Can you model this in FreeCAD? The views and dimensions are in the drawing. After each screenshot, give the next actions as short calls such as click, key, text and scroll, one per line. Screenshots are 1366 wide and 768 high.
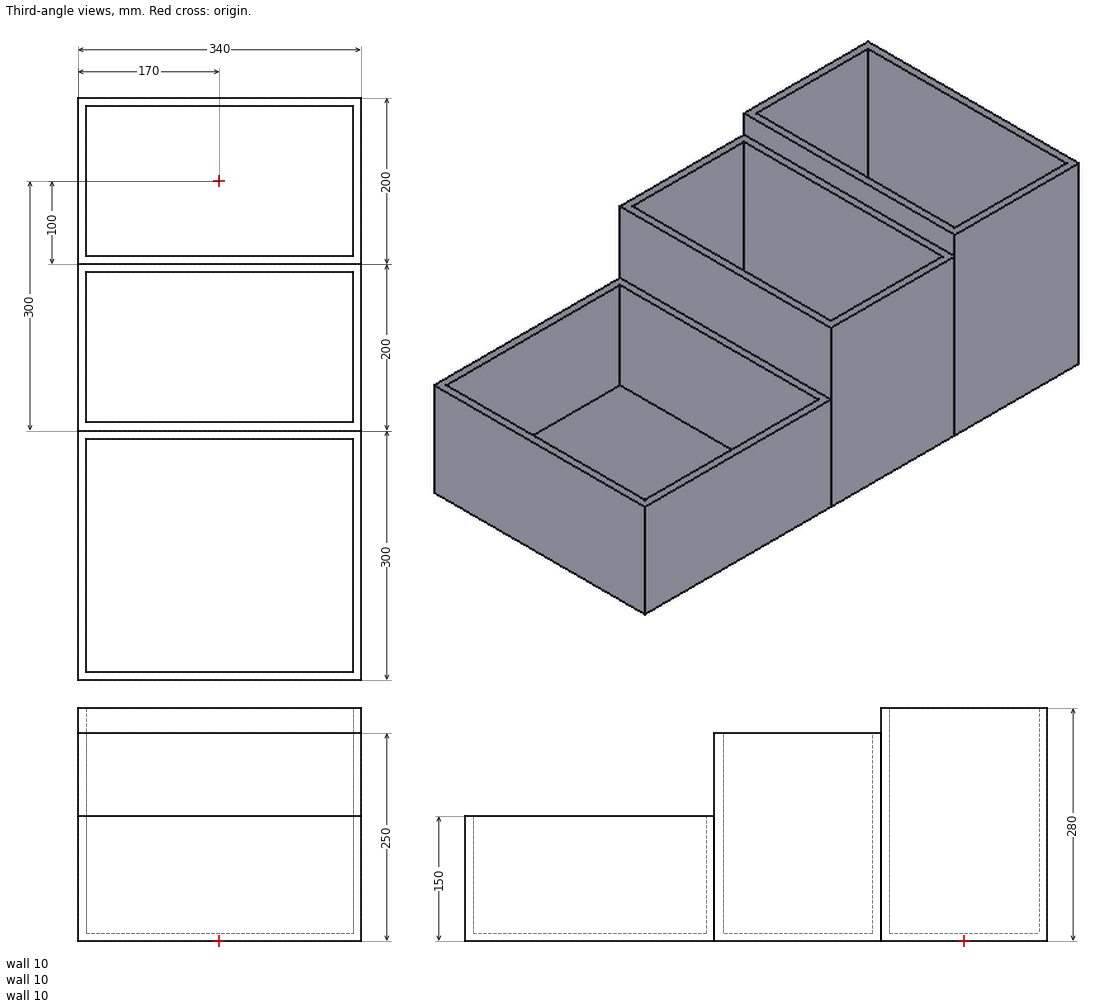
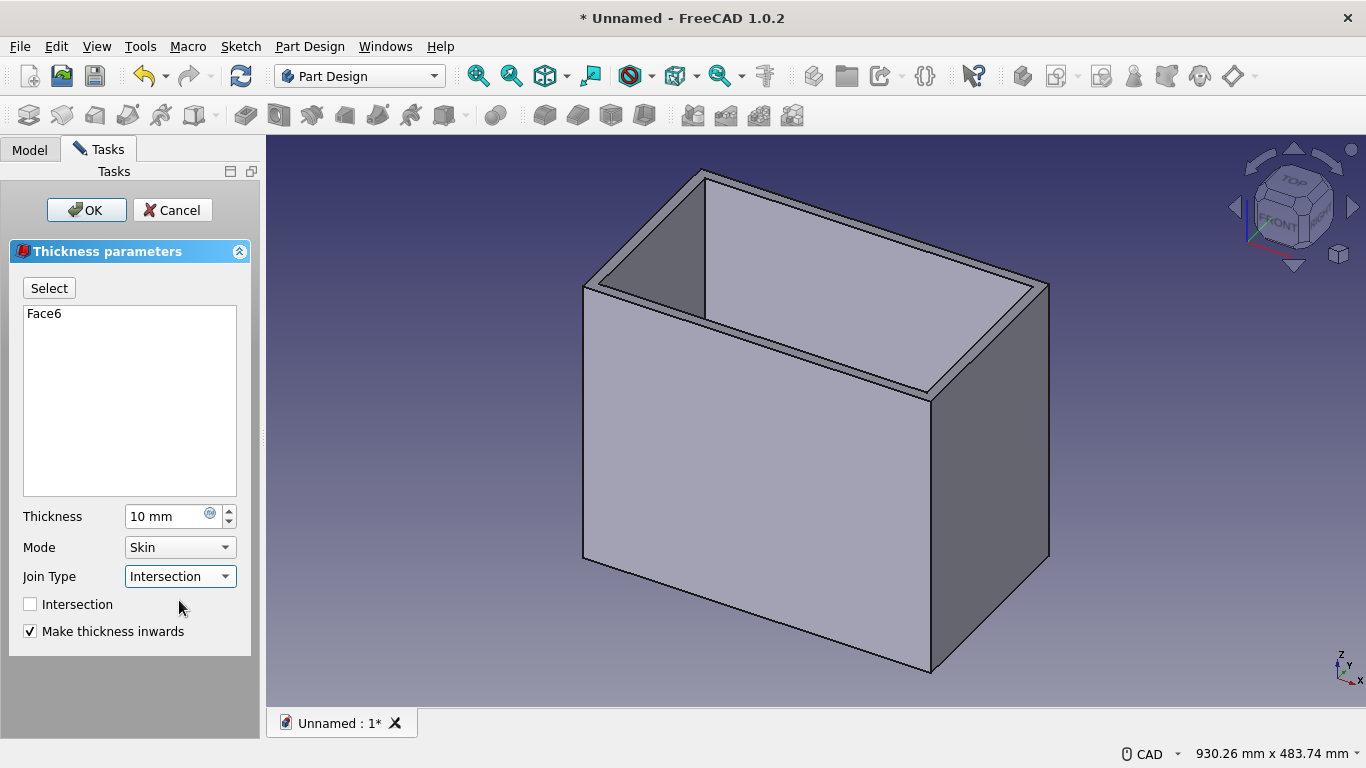
click(87, 210)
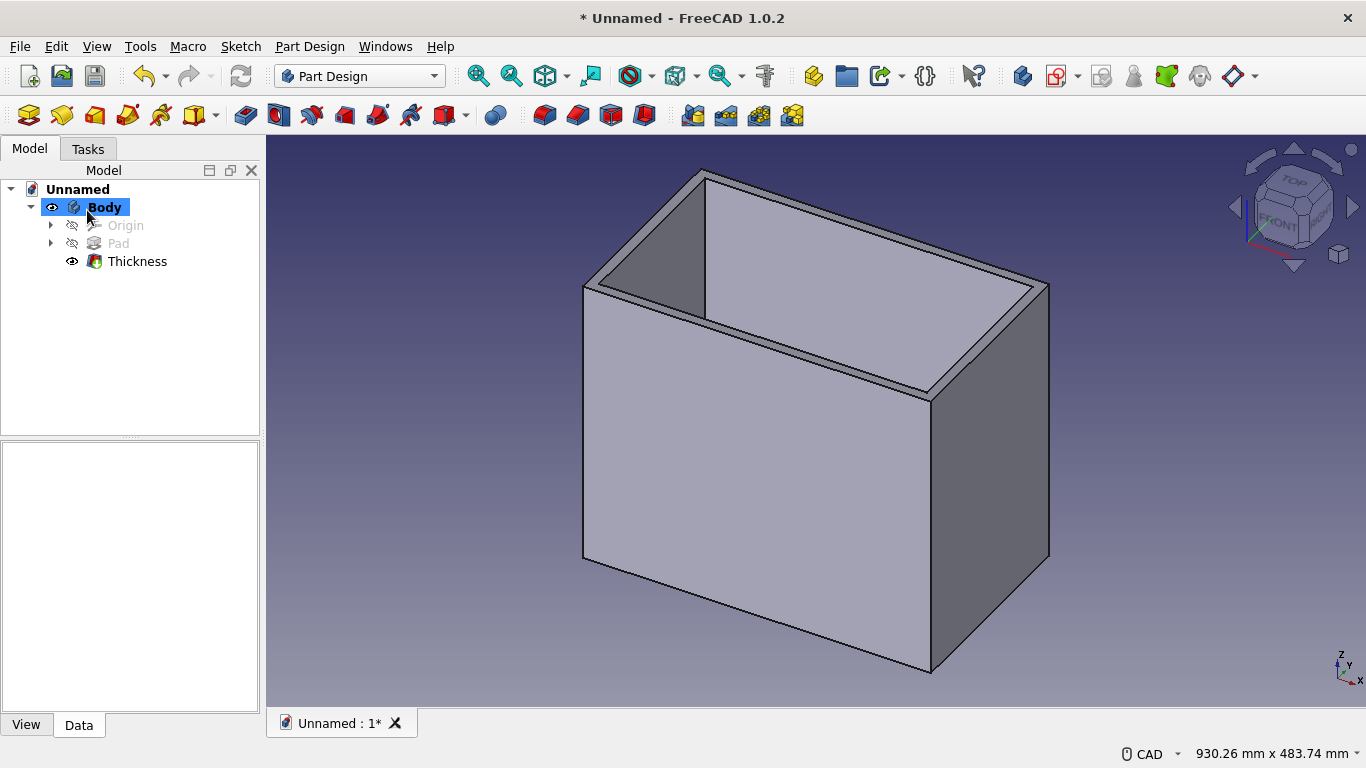
click(1023, 76)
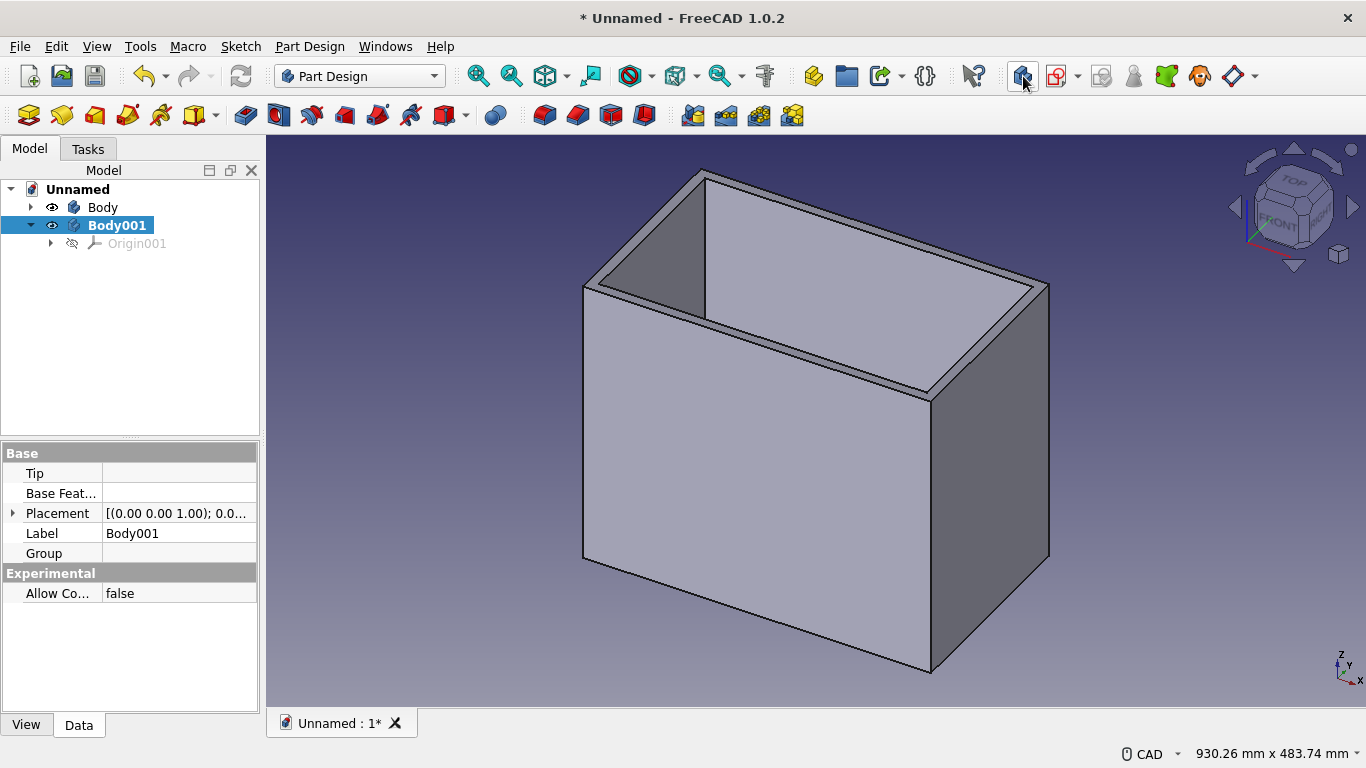
click(306, 667)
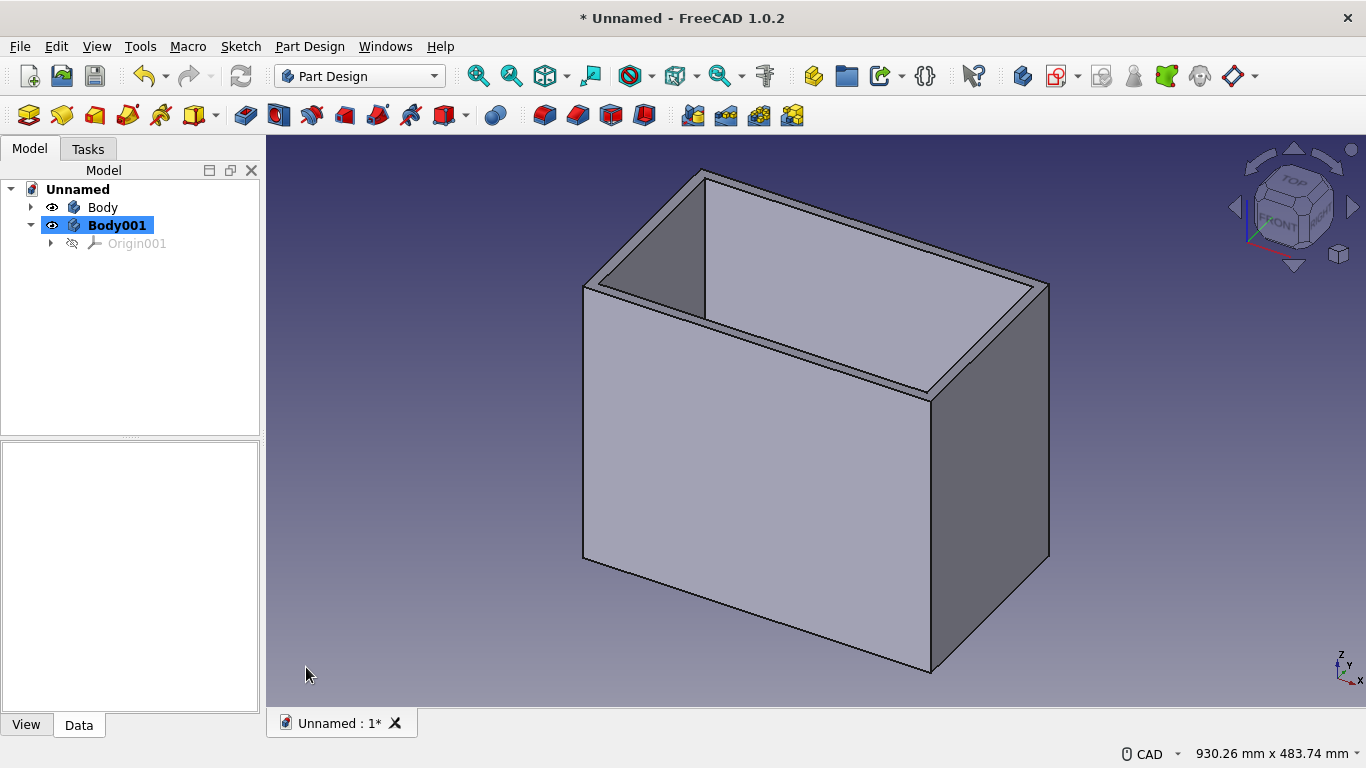
click(1056, 76)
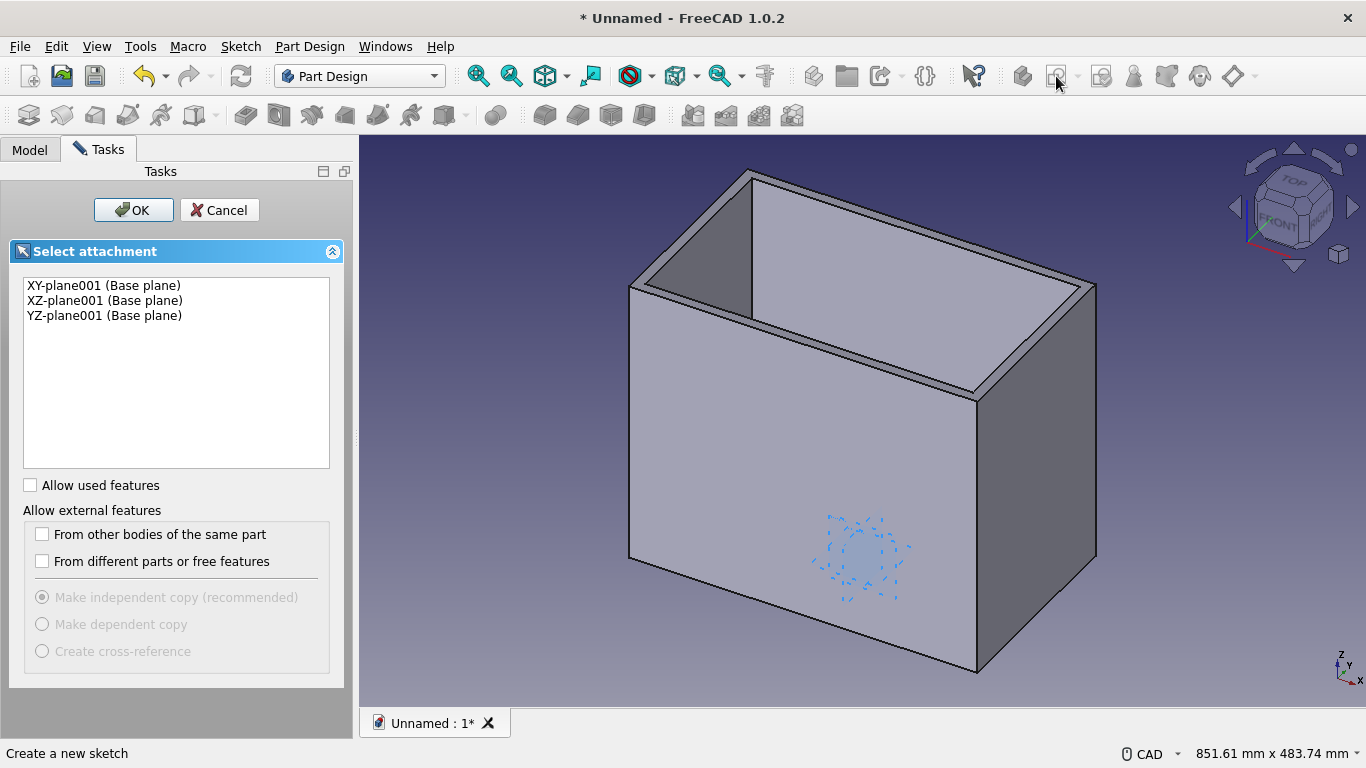
click(84, 286)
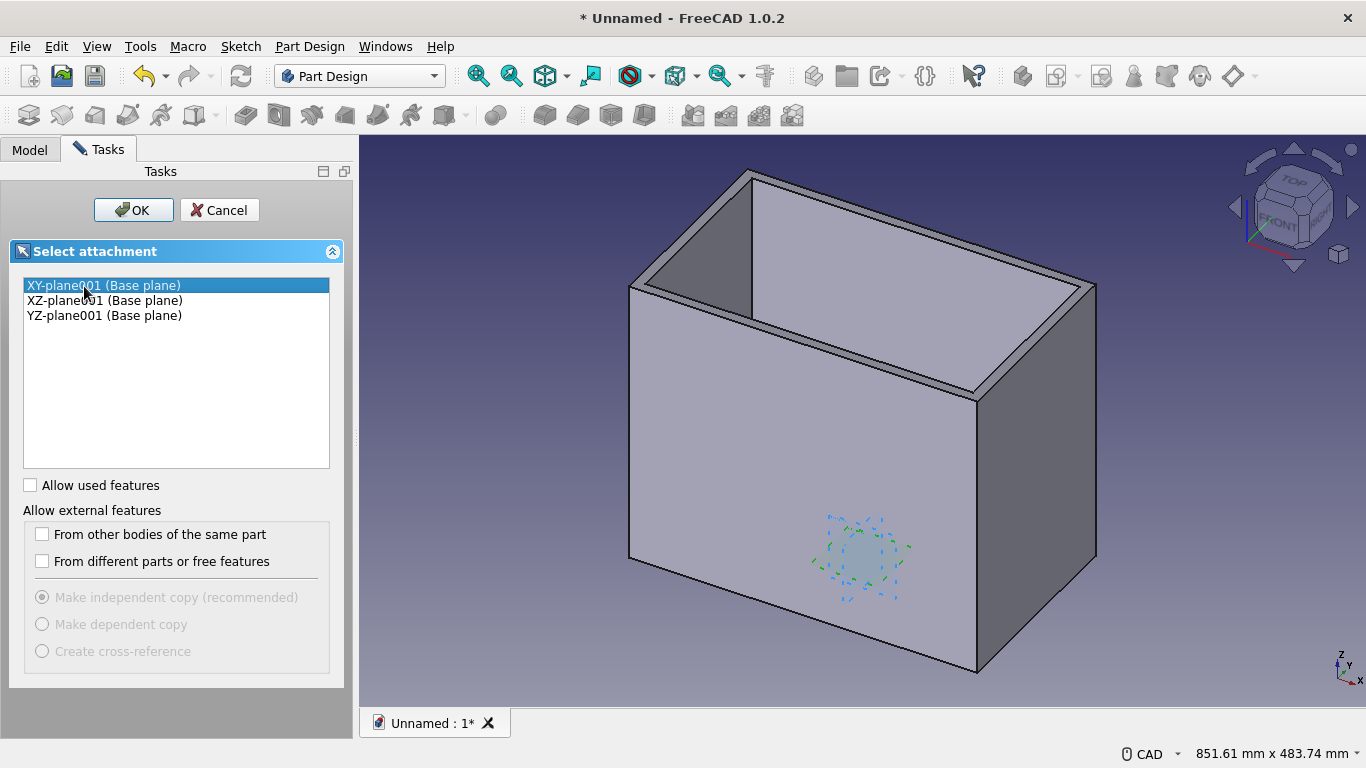
click(134, 210)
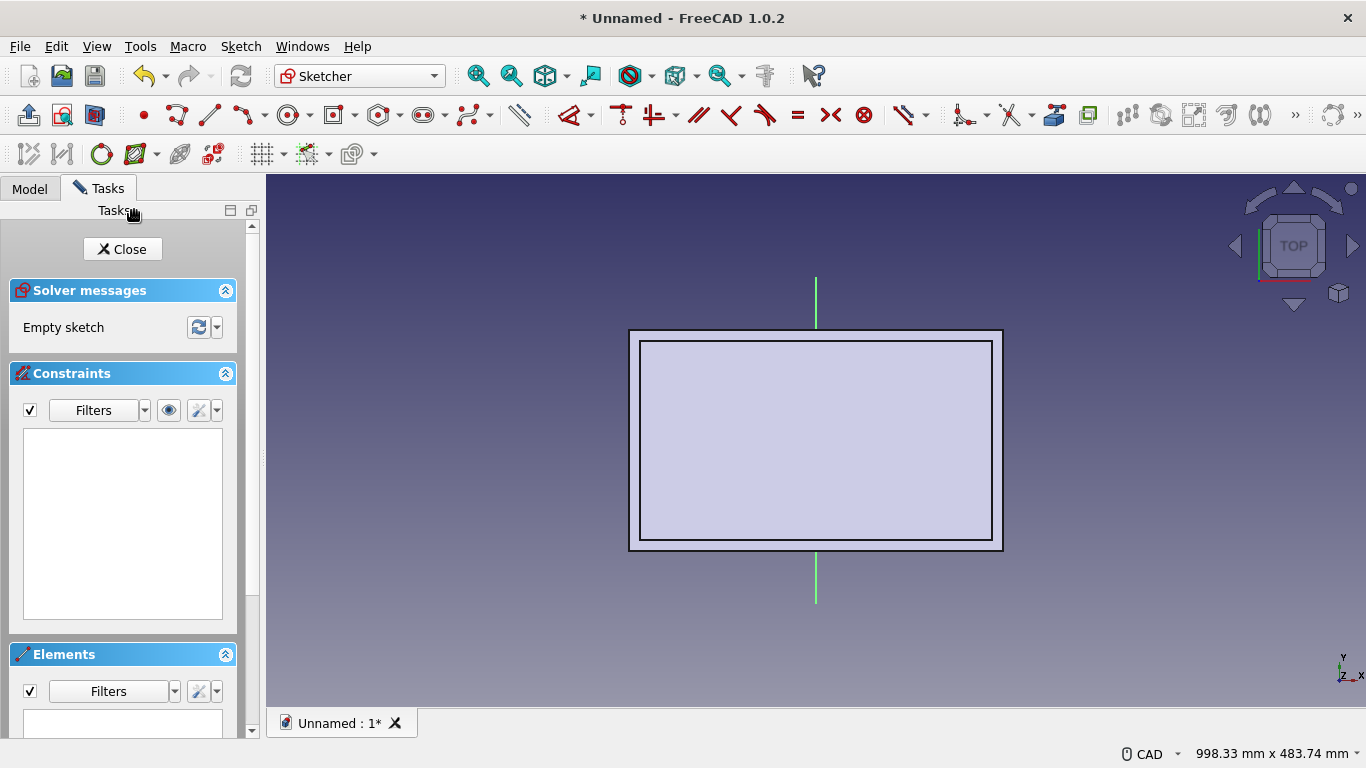
scroll(608, 202, down, 2)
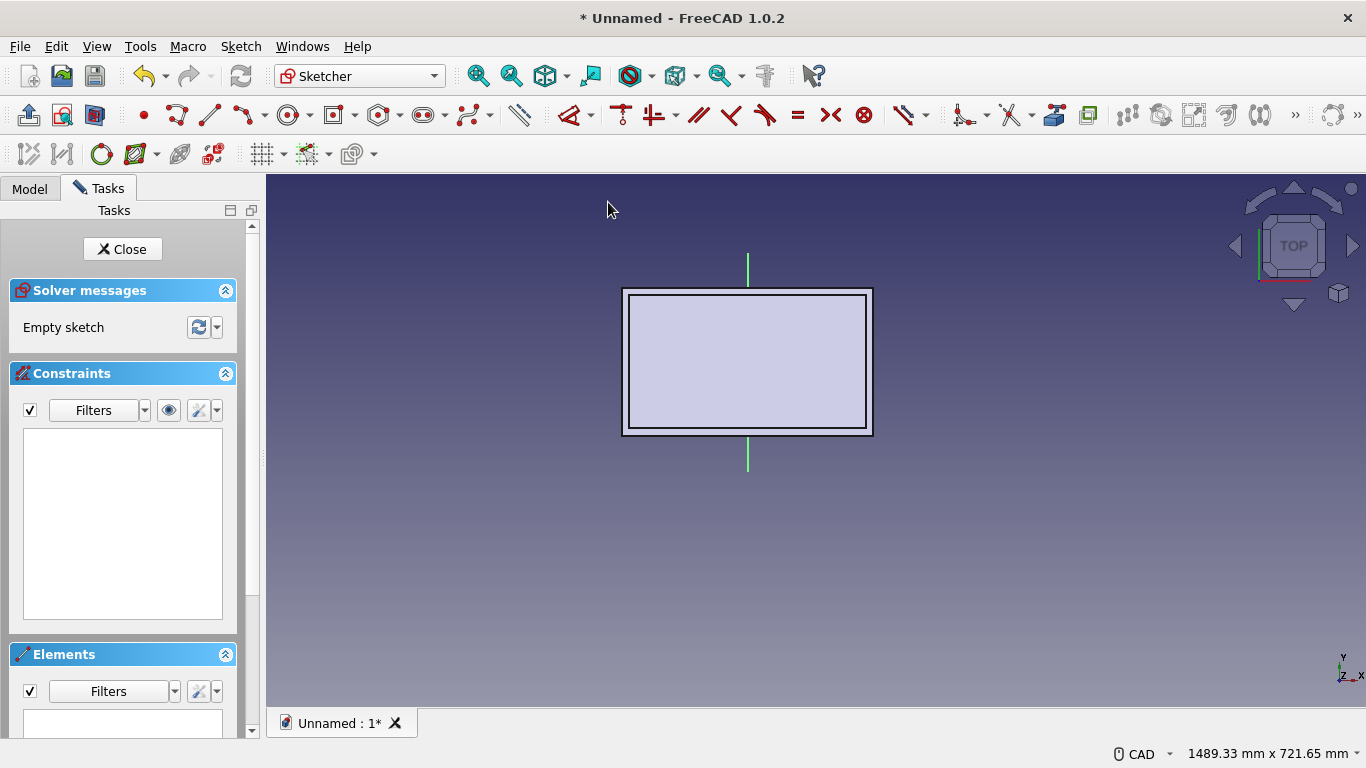
scroll(748, 538, up, 2)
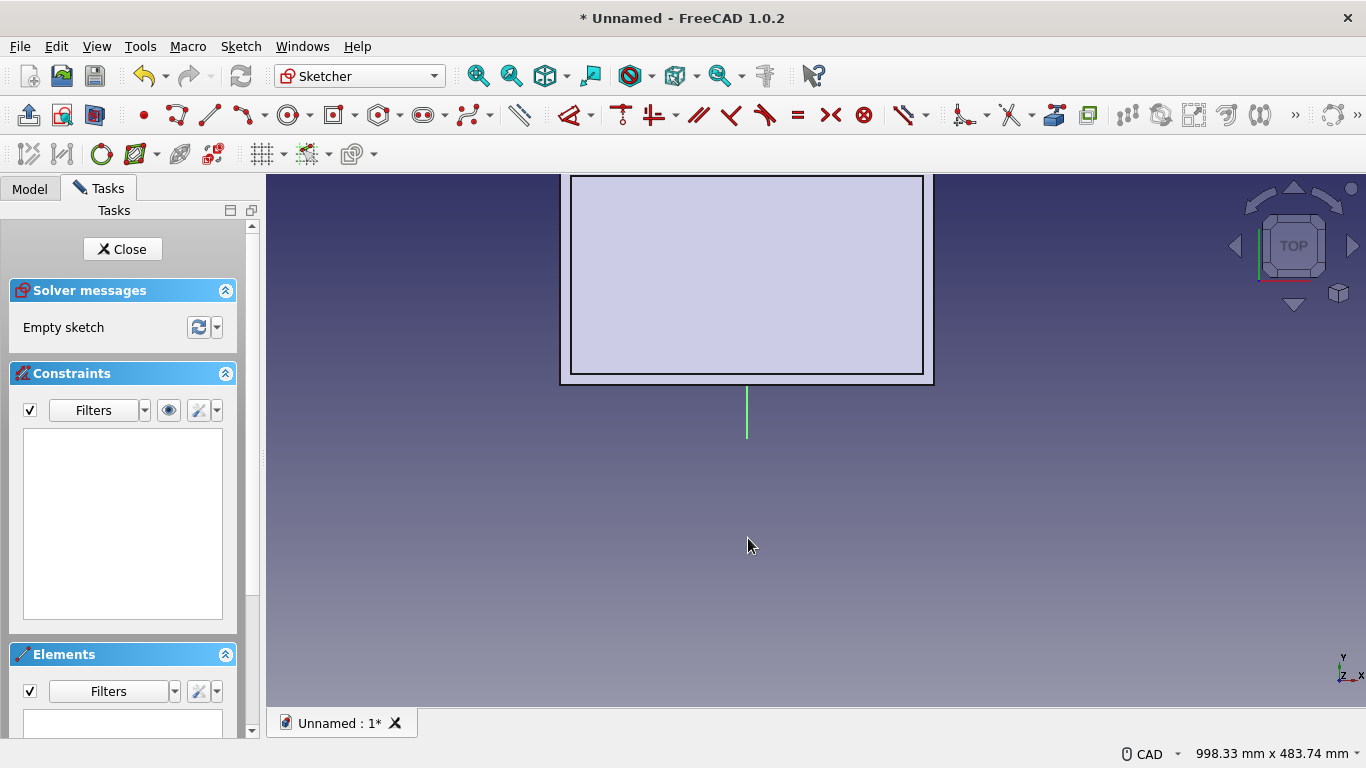
key(g)
key(r)